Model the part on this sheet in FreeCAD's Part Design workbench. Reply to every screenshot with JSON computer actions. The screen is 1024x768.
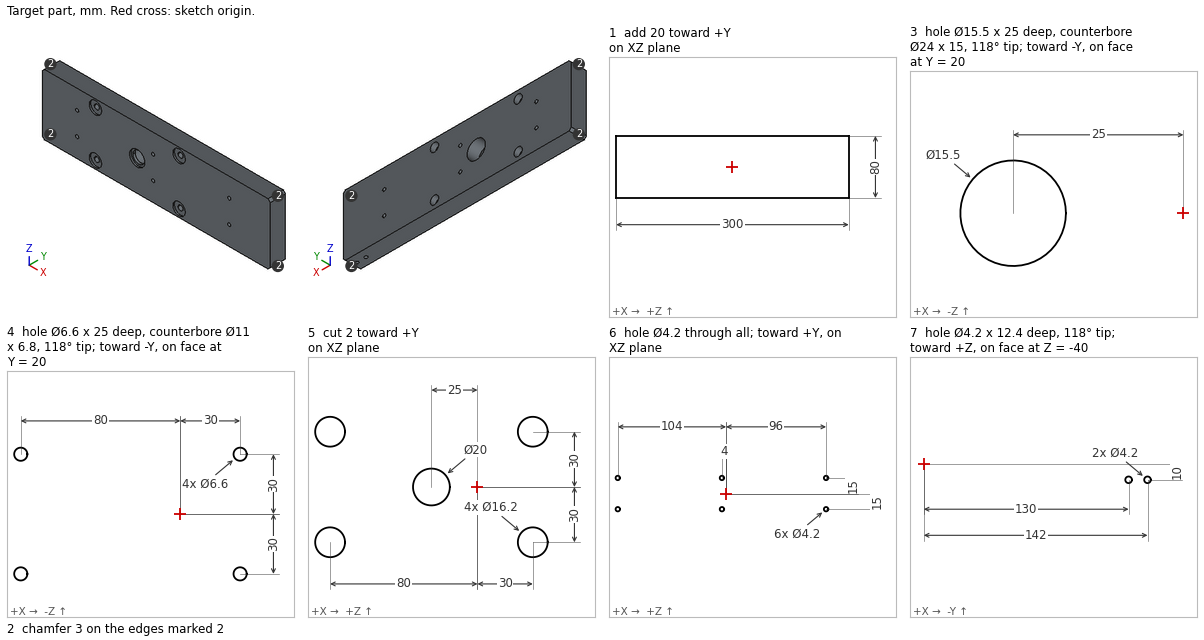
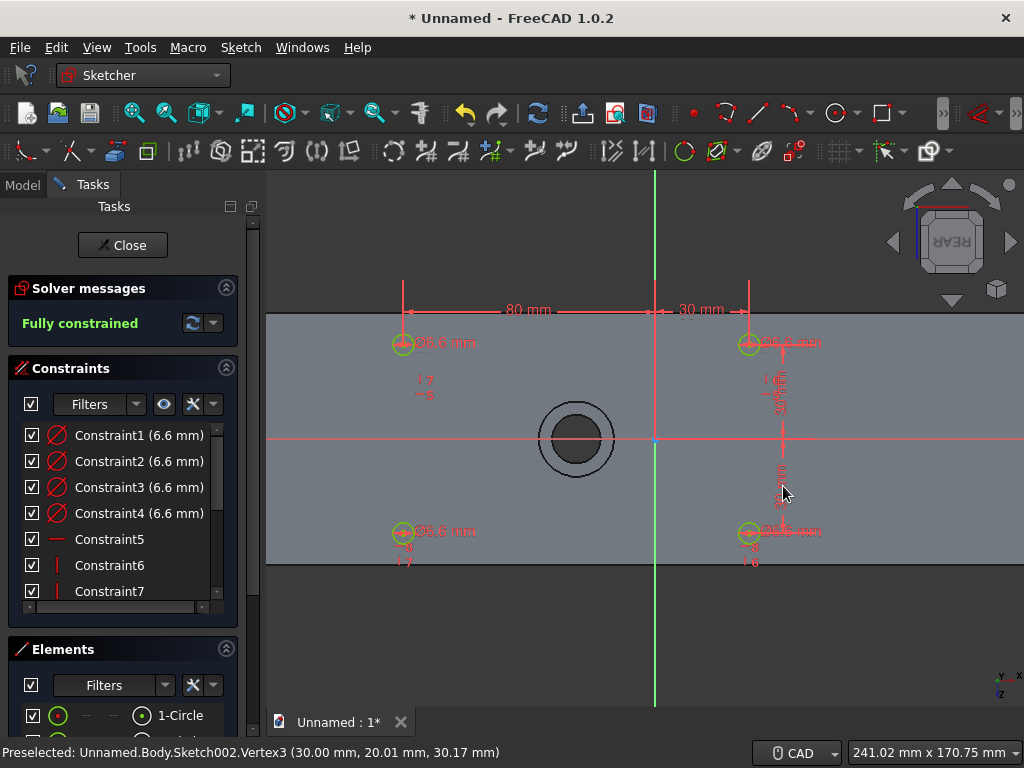
{"action": "left_click", "coordinate": [123, 245]}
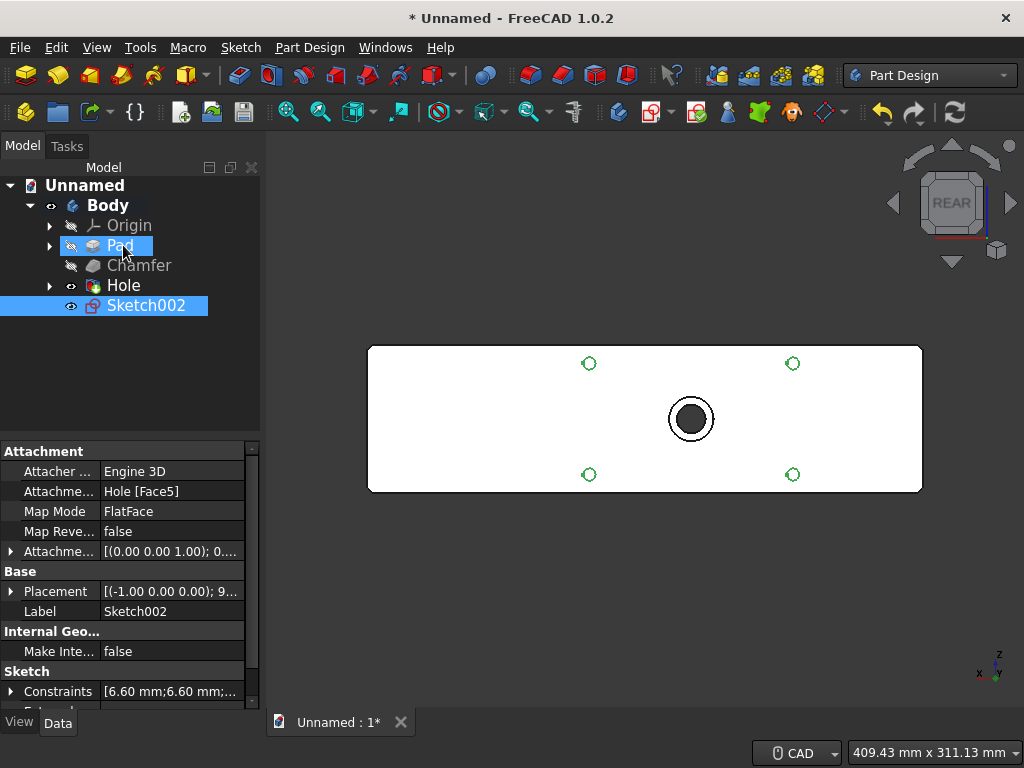
{"action": "left_click", "coordinate": [272, 76]}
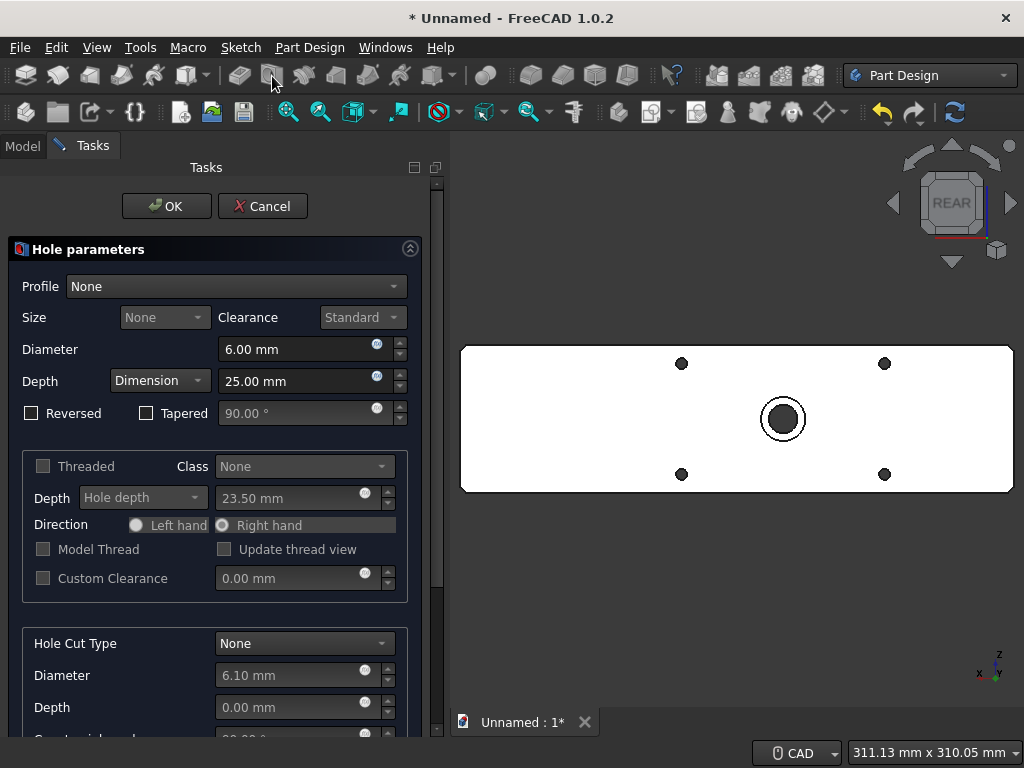
{"action": "triple_click", "coordinate": [305, 349]}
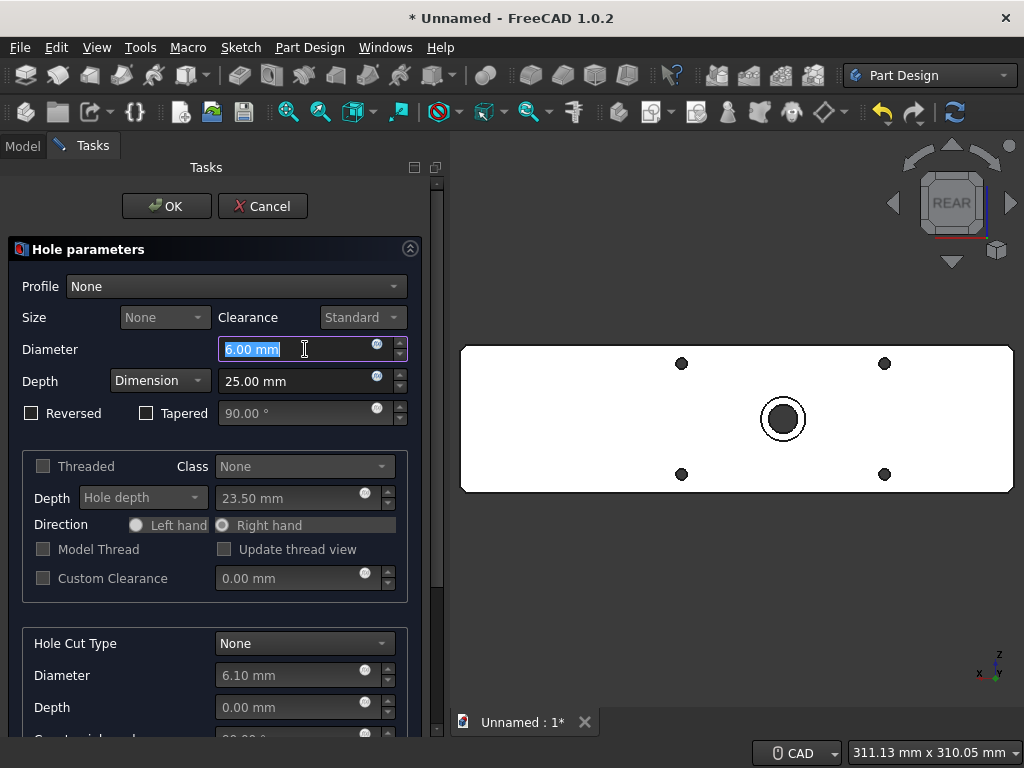
{"action": "type", "text": "6.6"}
{"action": "key", "text": "Tab"}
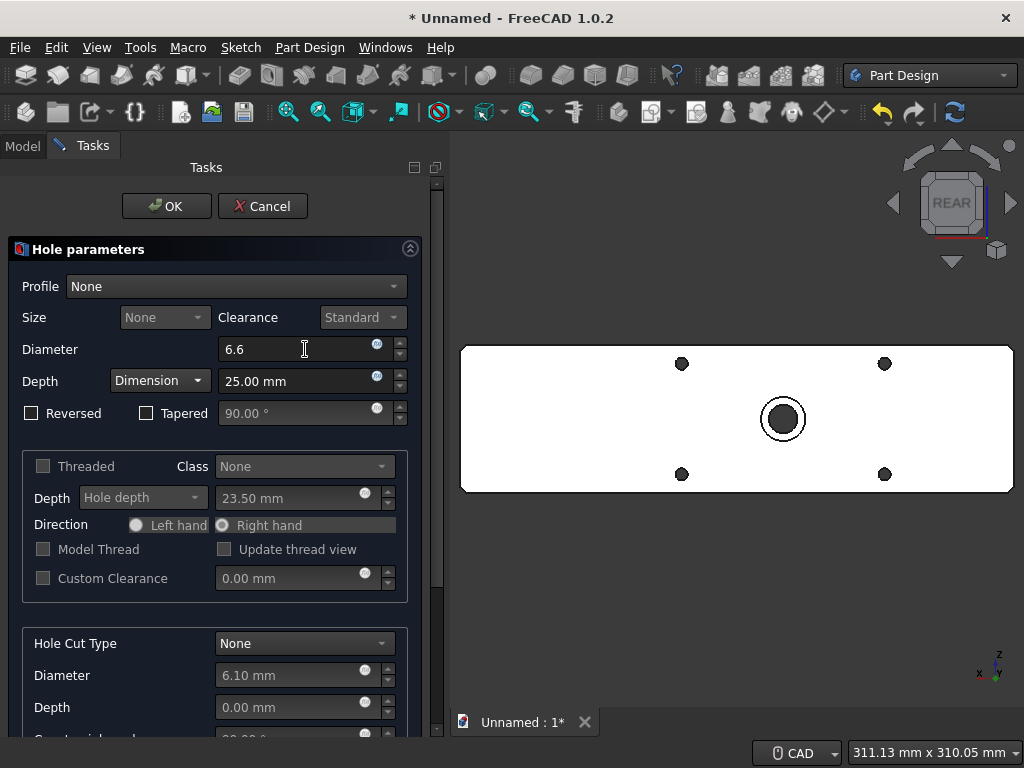
{"action": "triple_click", "coordinate": [305, 381]}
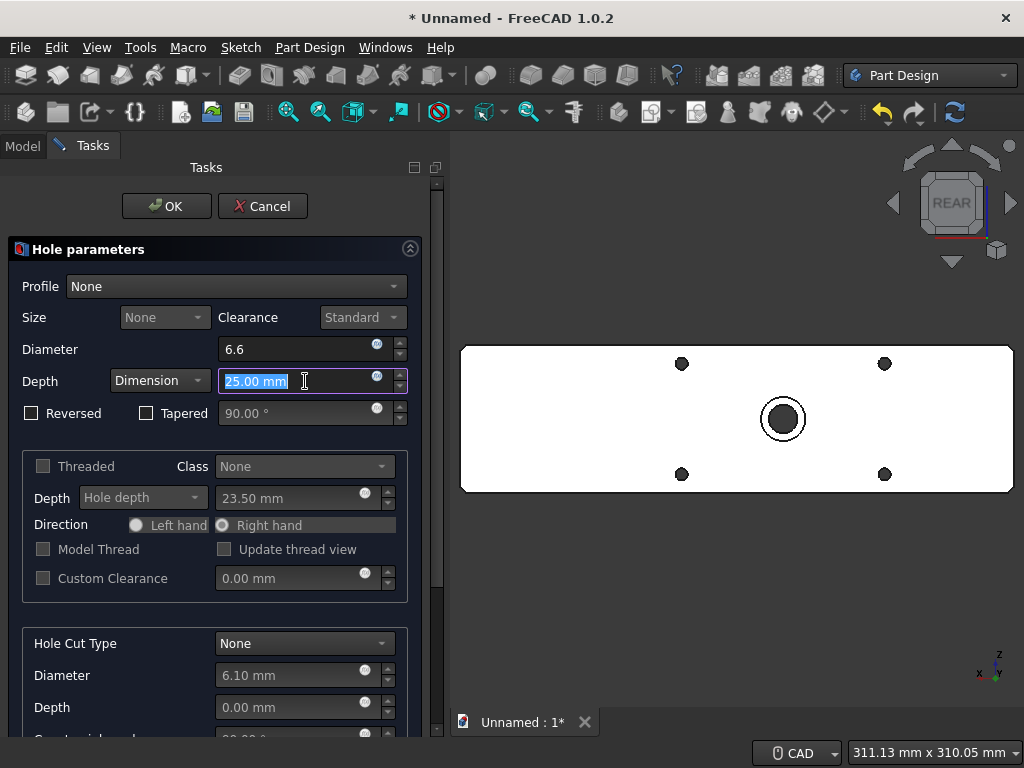
{"action": "type", "text": "25"}
{"action": "key", "text": "Tab"}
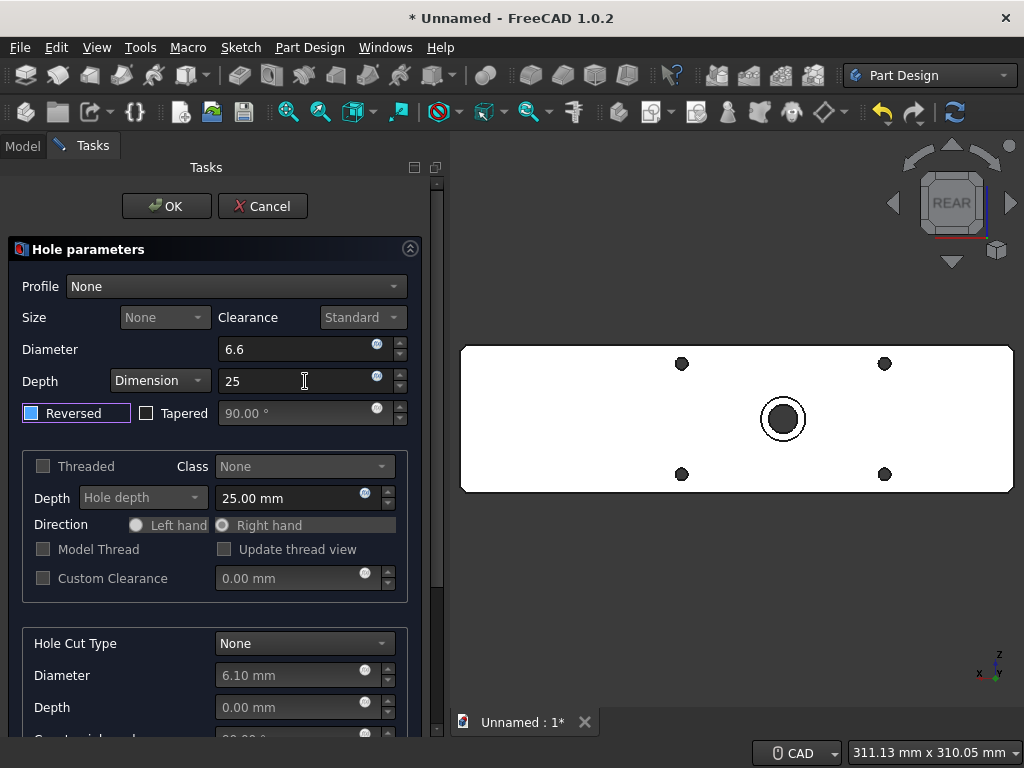
{"action": "left_click", "coordinate": [306, 644]}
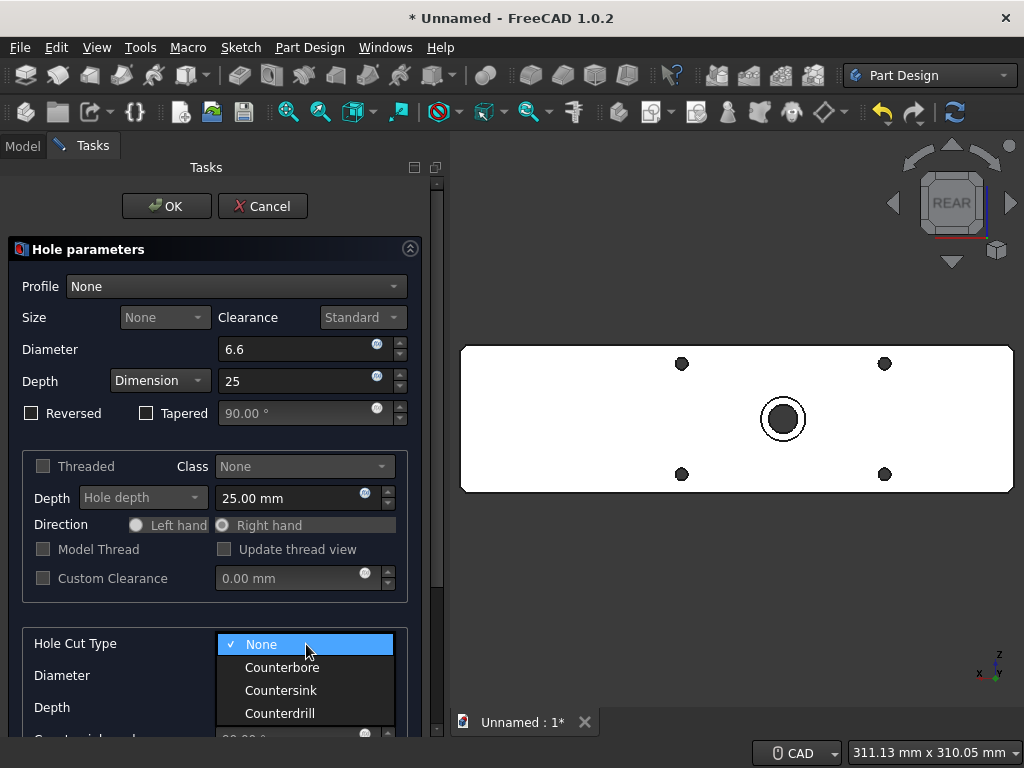
{"action": "left_click", "coordinate": [304, 668]}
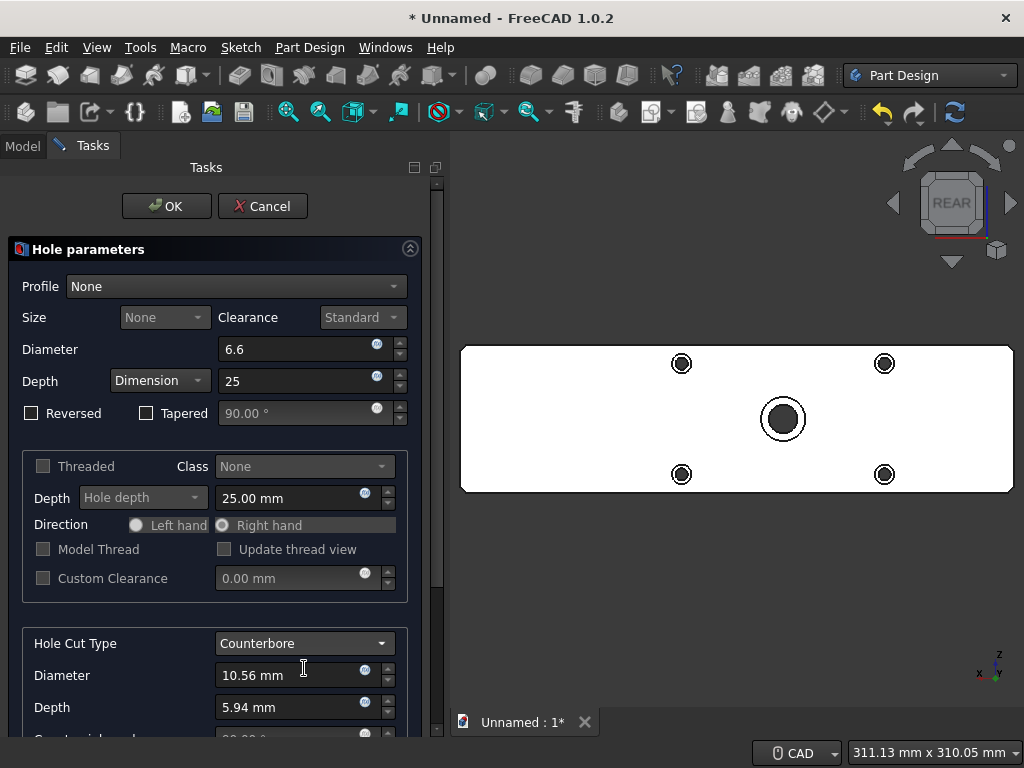
{"action": "triple_click", "coordinate": [298, 675]}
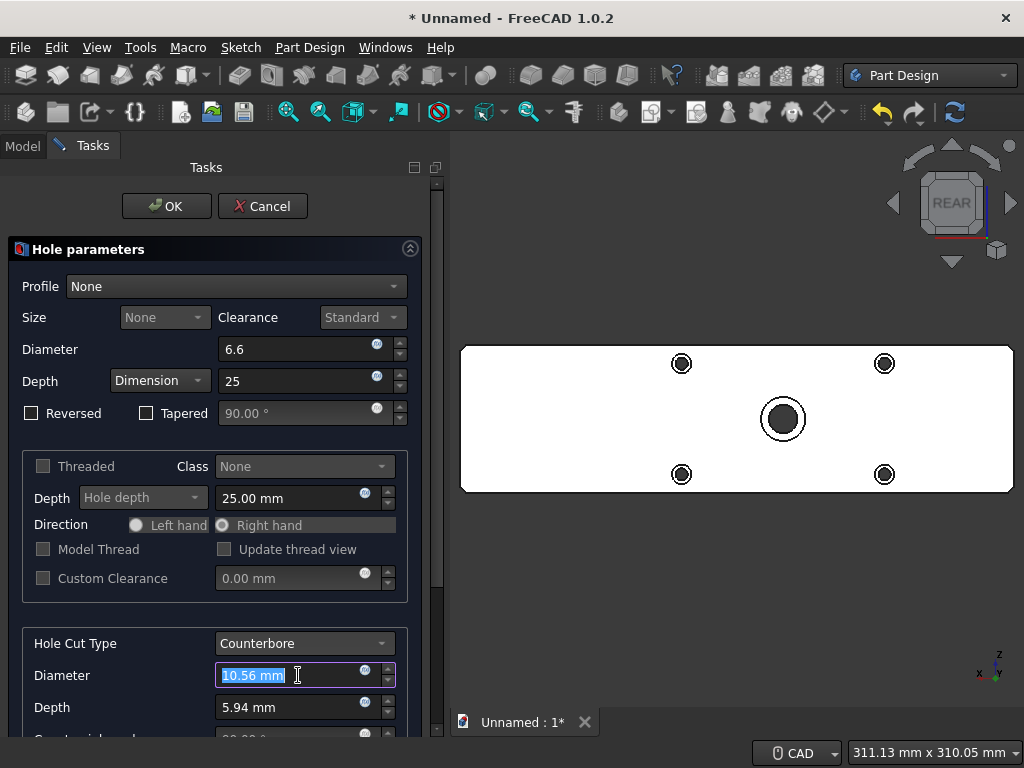
{"action": "type", "text": "11"}
{"action": "key", "text": "Tab"}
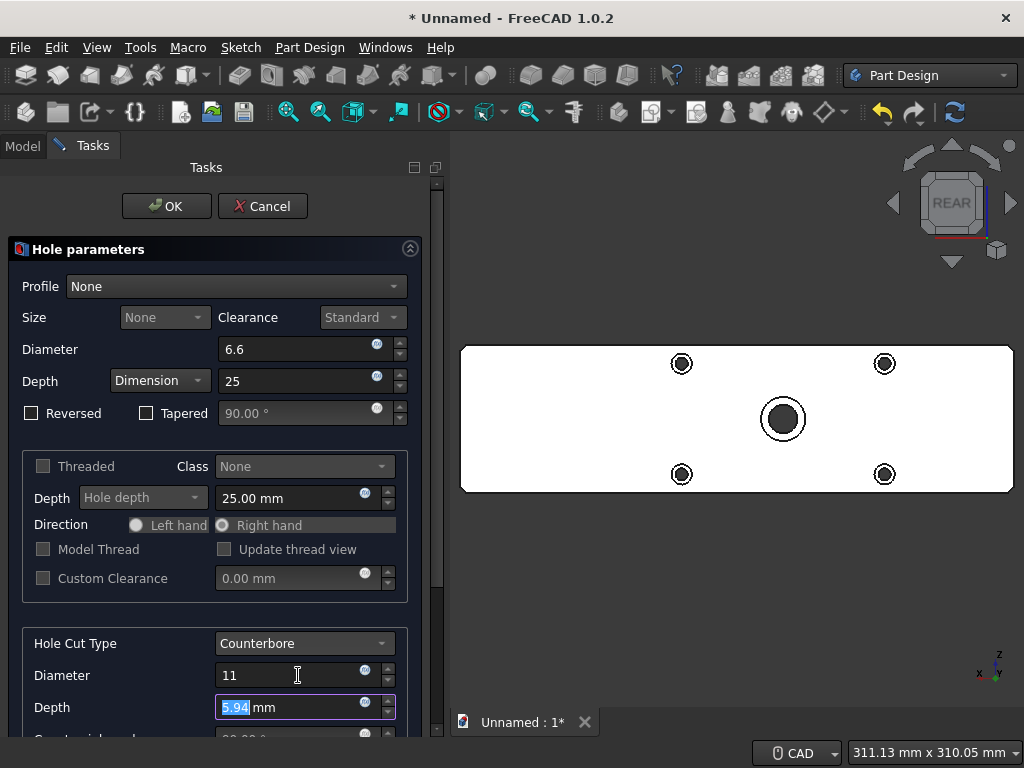
{"action": "type", "text": "6.8"}
{"action": "key", "text": "Tab"}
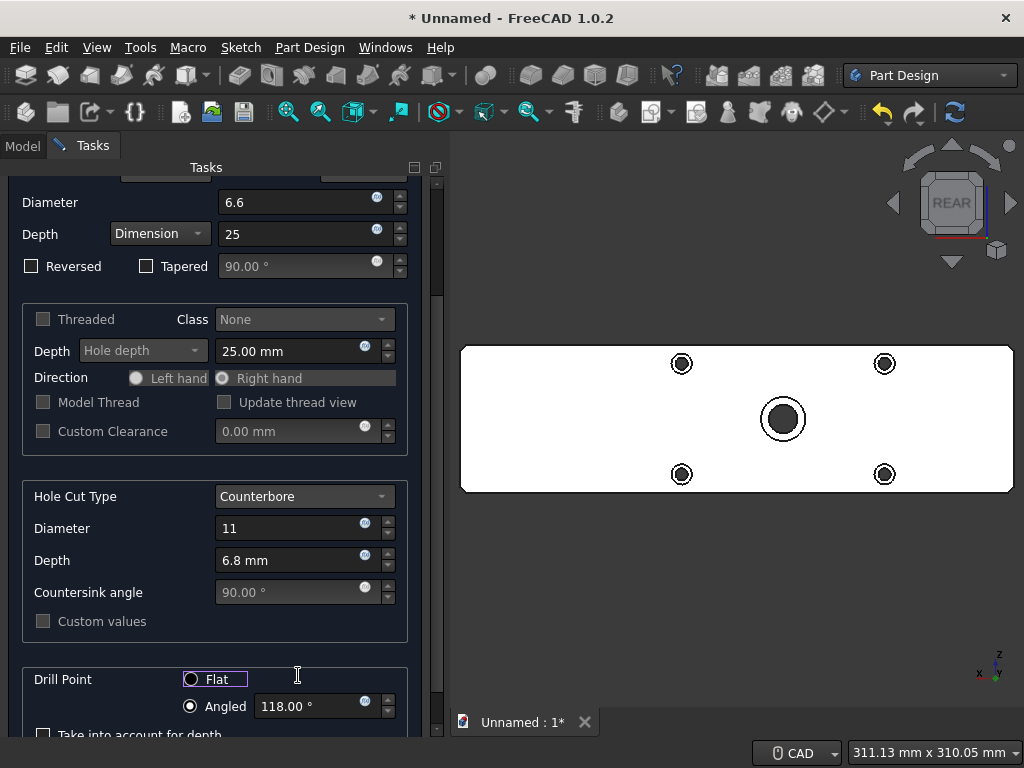
{"action": "scroll", "coordinate": [437, 456], "scroll_direction": "up", "scroll_amount": 4}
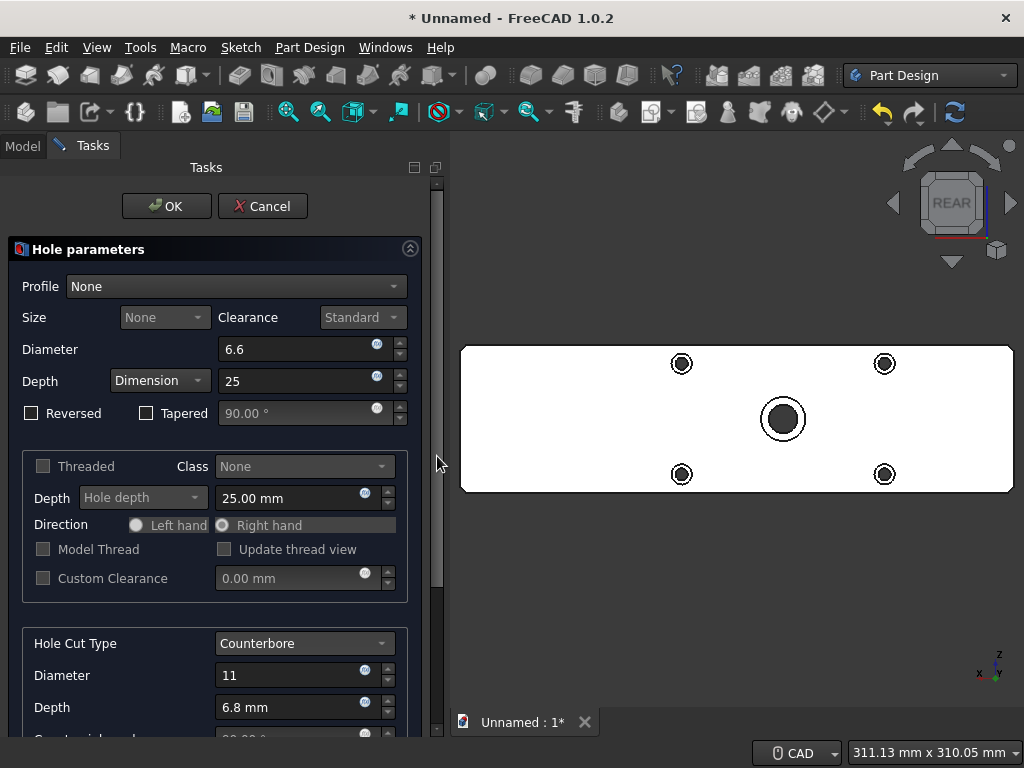
{"action": "left_click", "coordinate": [167, 206]}